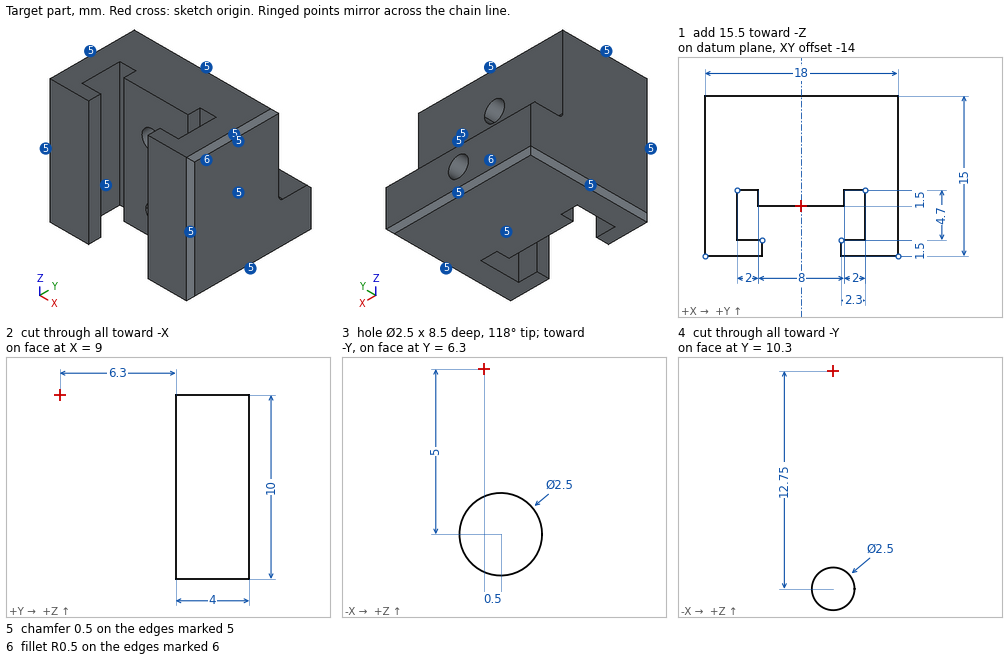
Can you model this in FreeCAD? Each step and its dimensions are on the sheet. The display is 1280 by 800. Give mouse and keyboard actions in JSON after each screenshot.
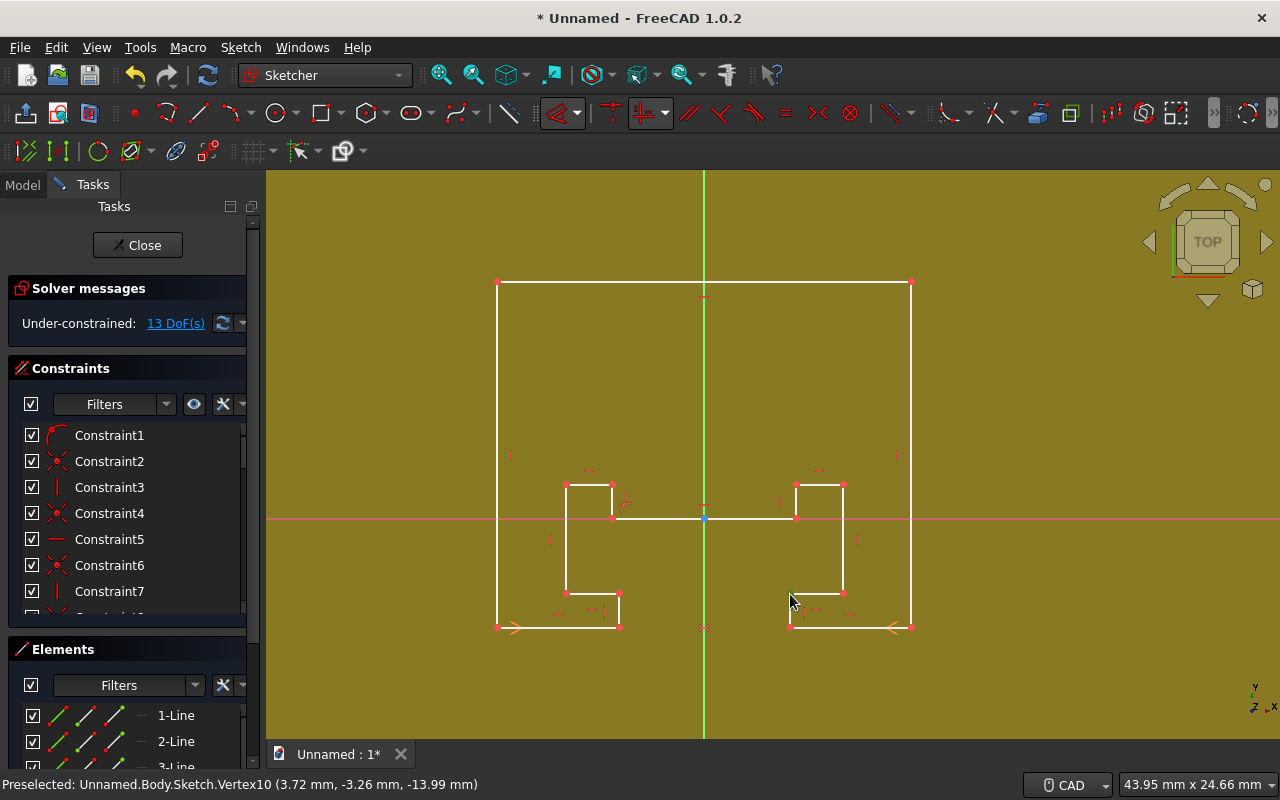
{"action": "left_click", "coordinate": [619, 594]}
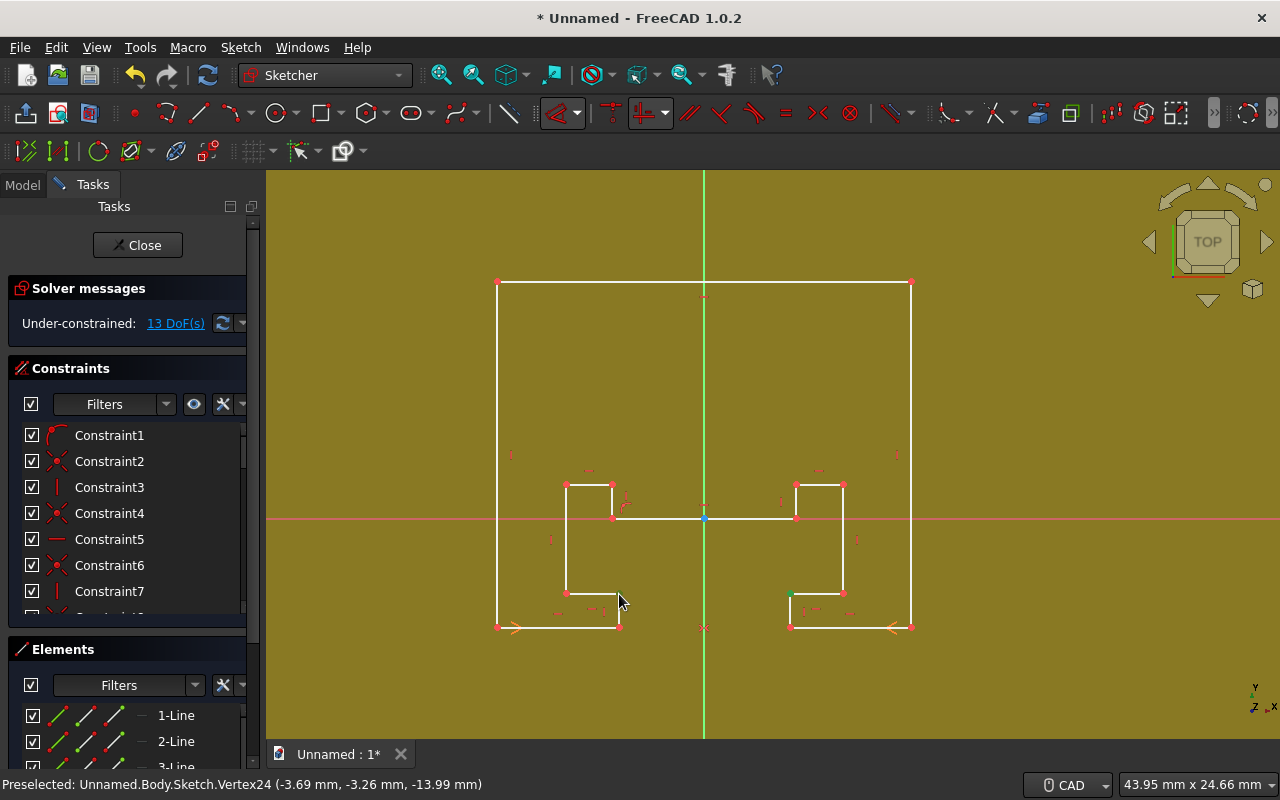
{"action": "left_click", "coordinate": [704, 674]}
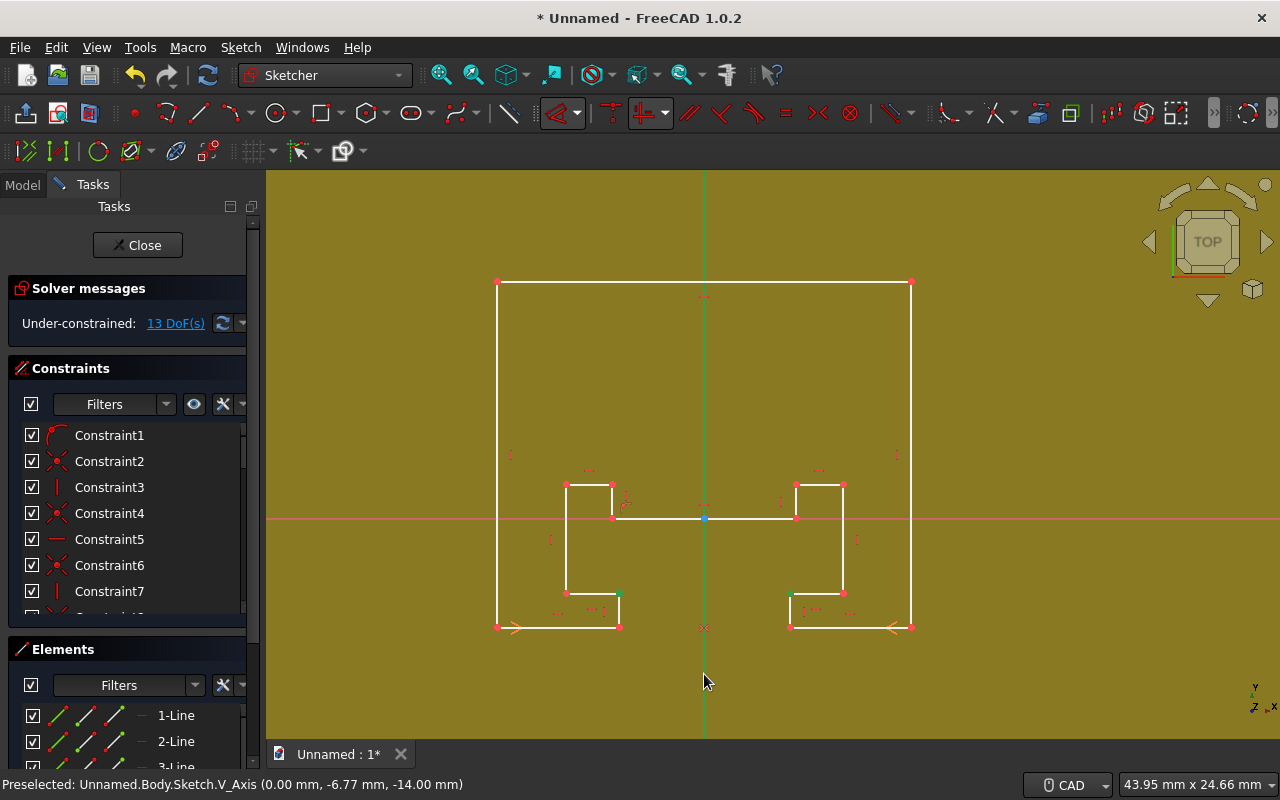
{"action": "key", "text": "s"}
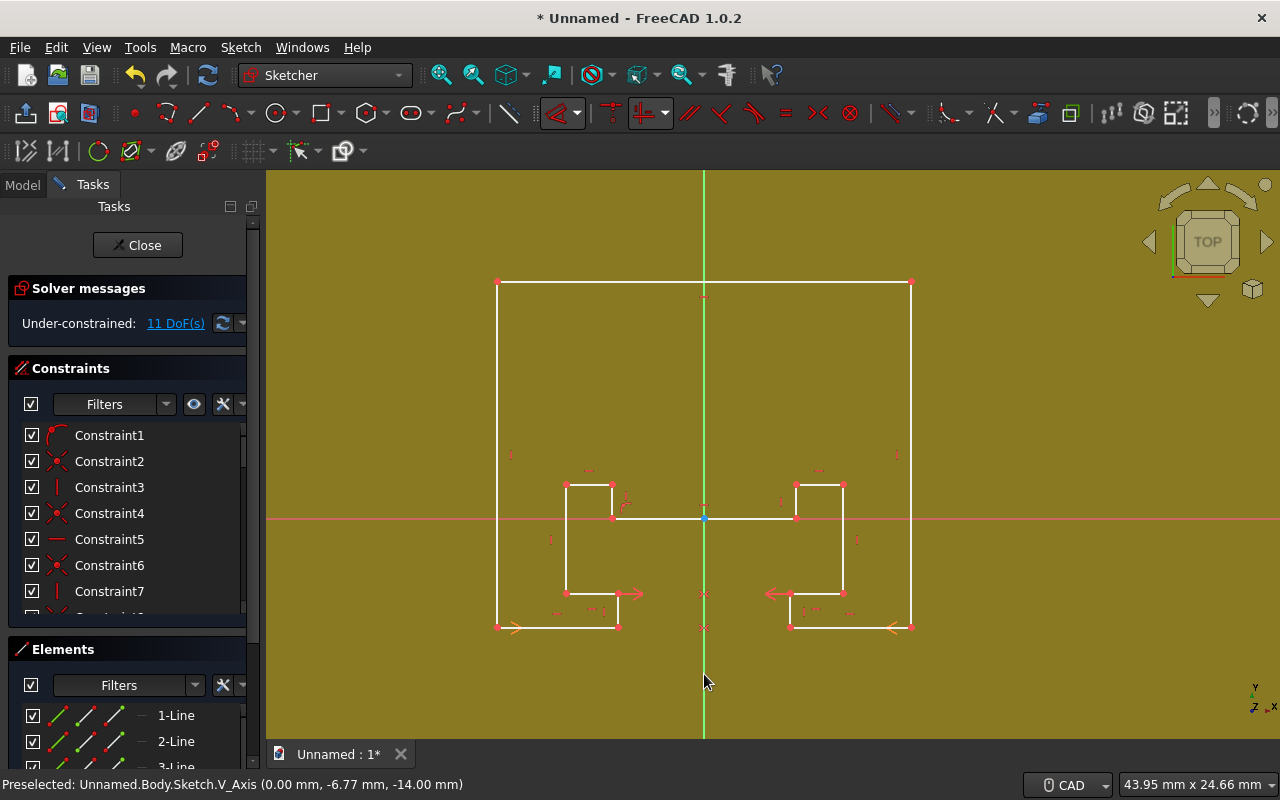
{"action": "left_click", "coordinate": [843, 485]}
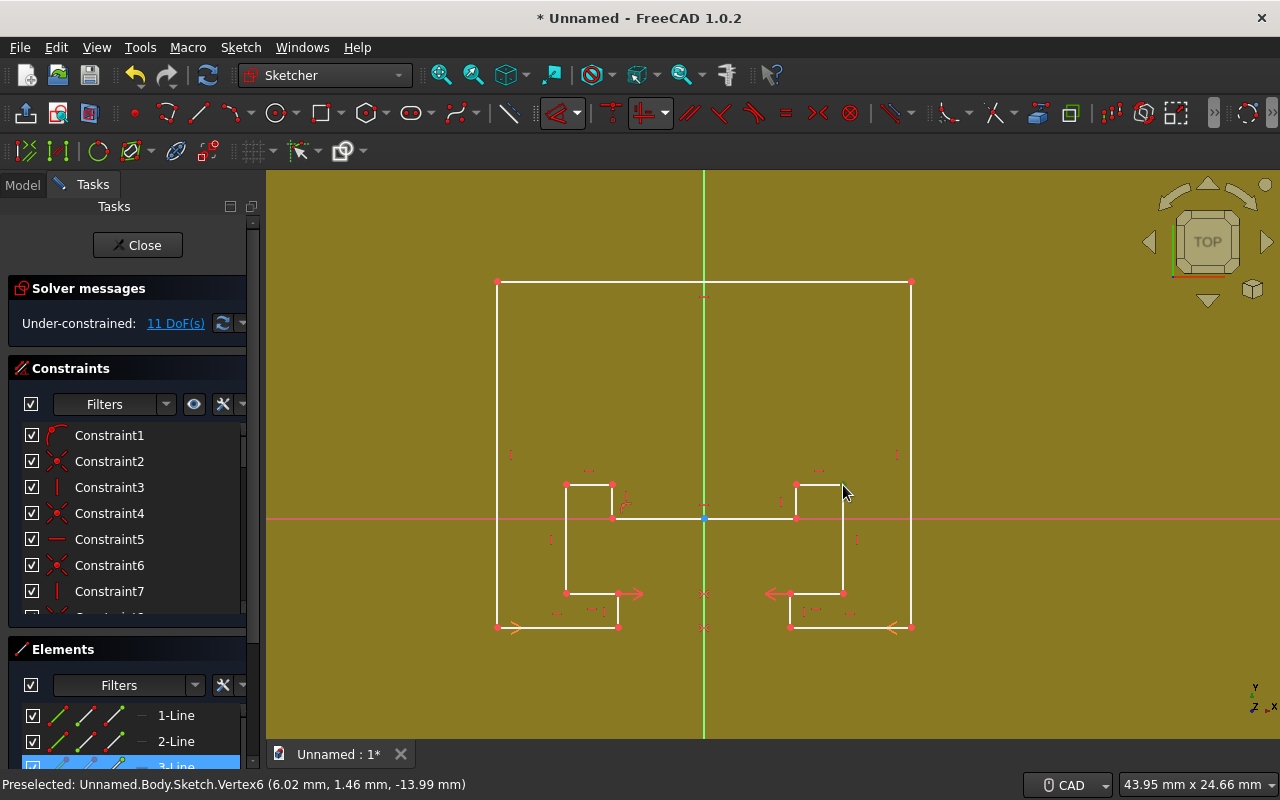
{"action": "left_click", "coordinate": [566, 485]}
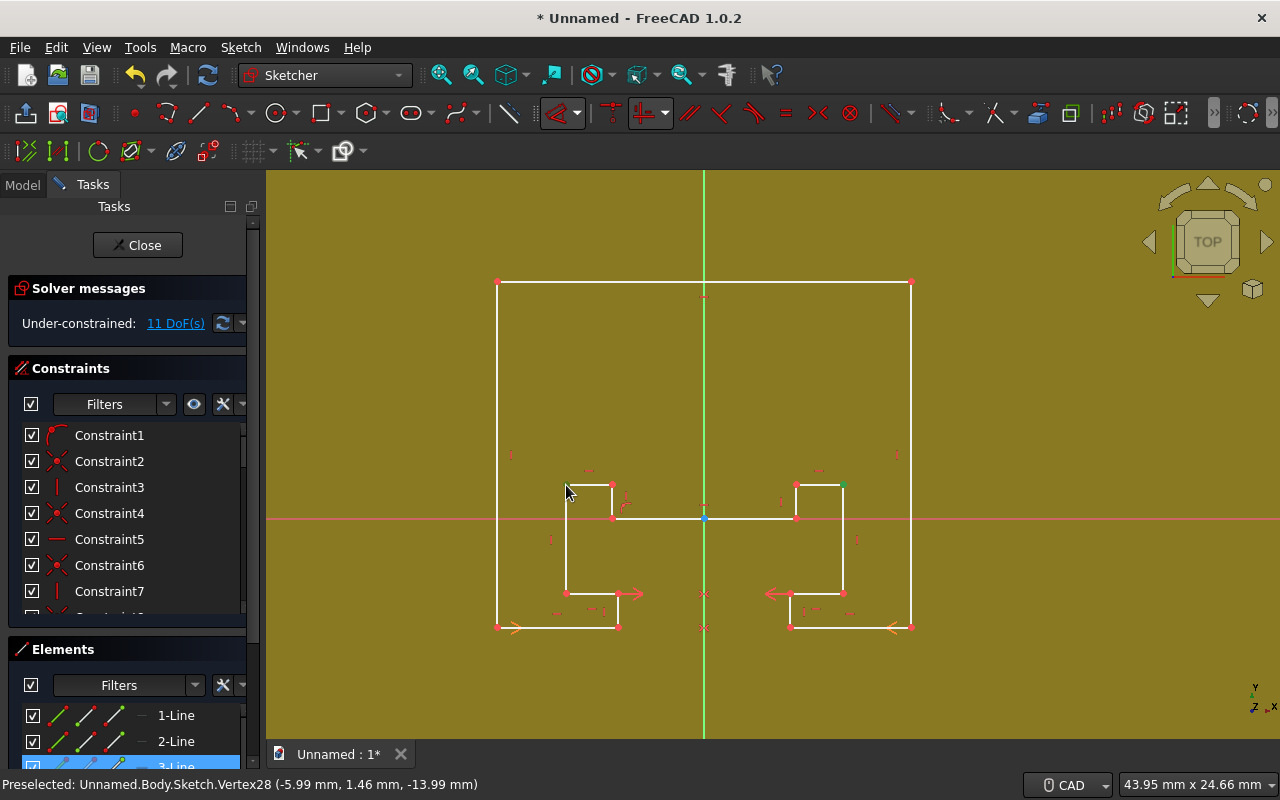
{"action": "left_click", "coordinate": [704, 674]}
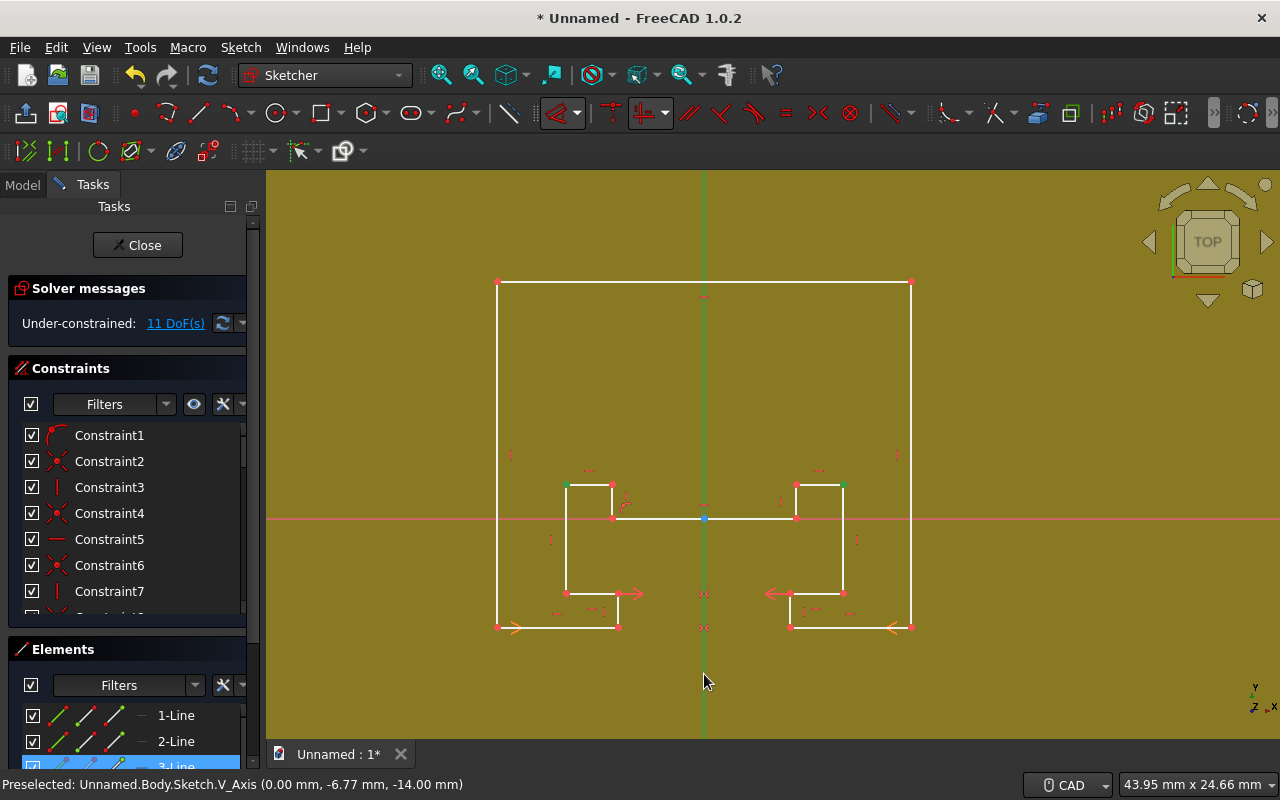
{"action": "left_click", "coordinate": [818, 114]}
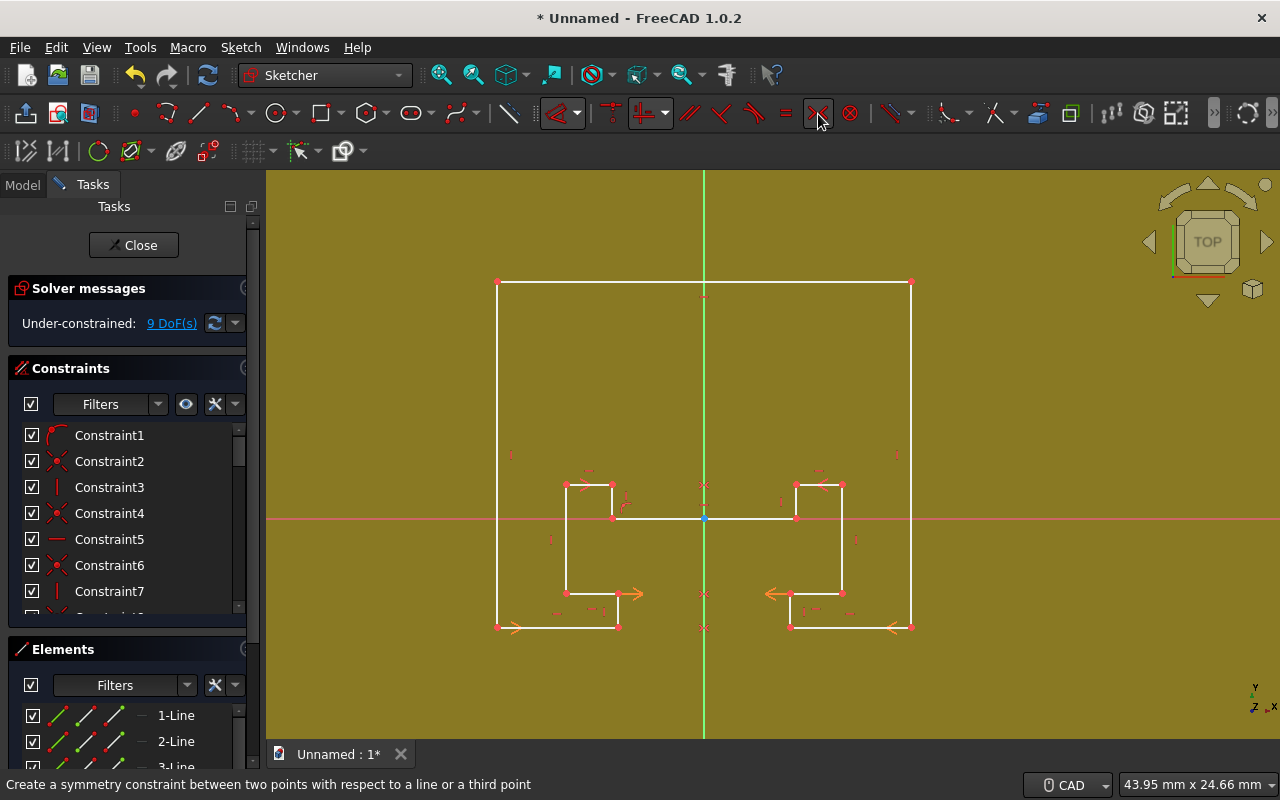
{"action": "key", "text": "d"}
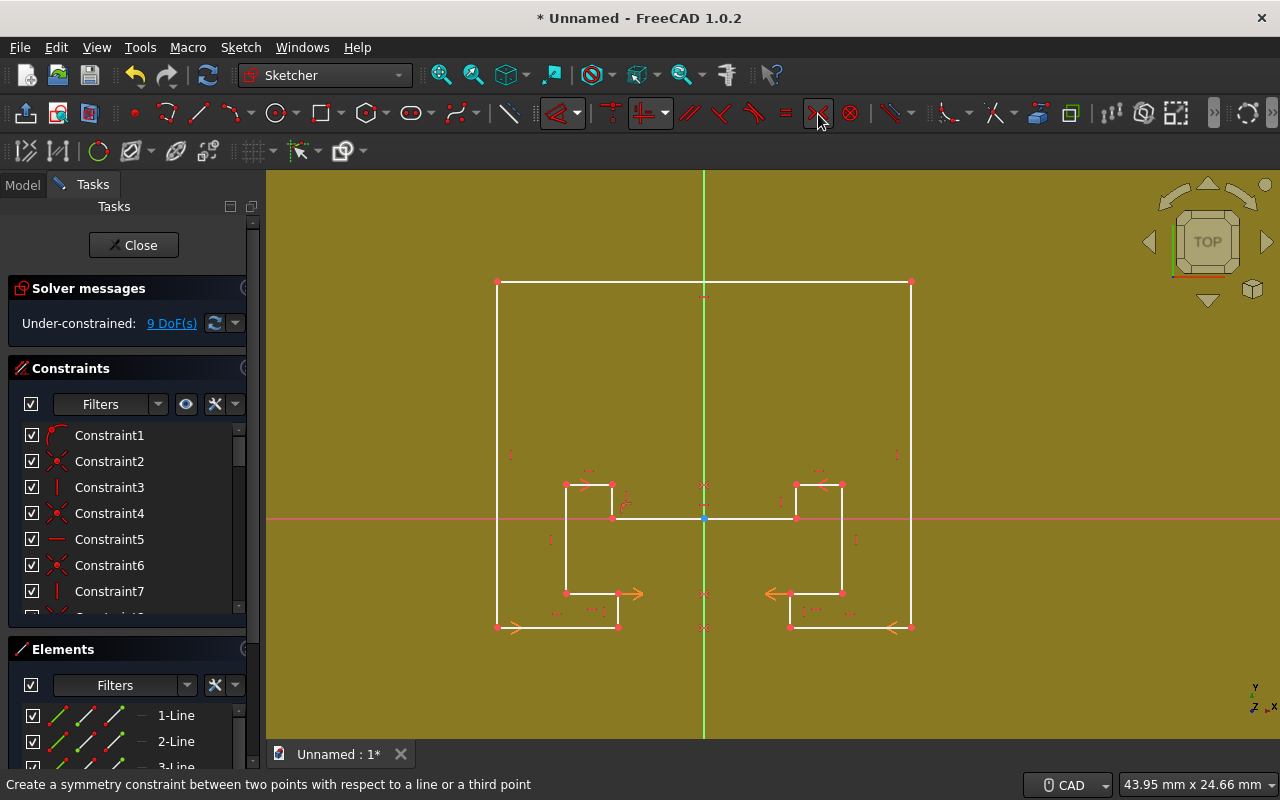
{"action": "left_click", "coordinate": [667, 519]}
{"action": "left_click", "coordinate": [662, 553]}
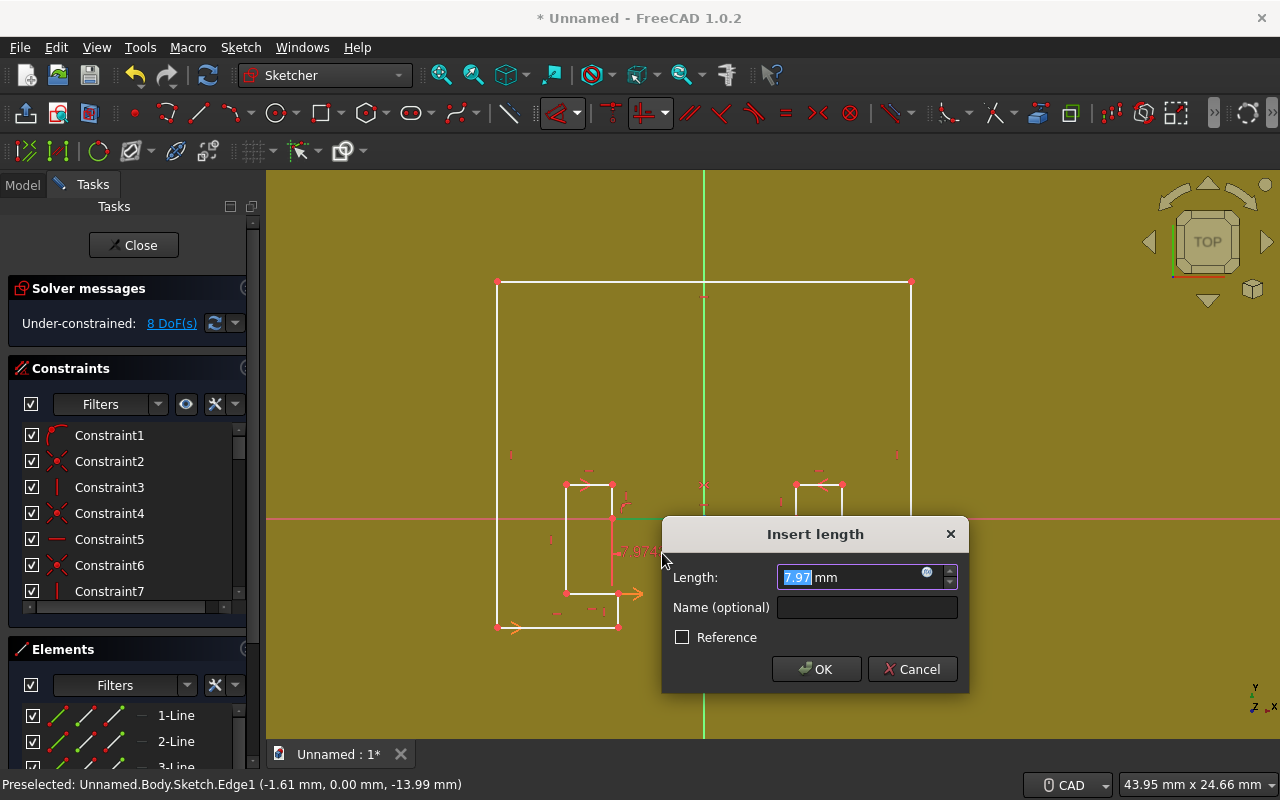
{"action": "type", "text": "8"}
{"action": "key", "text": "Return"}